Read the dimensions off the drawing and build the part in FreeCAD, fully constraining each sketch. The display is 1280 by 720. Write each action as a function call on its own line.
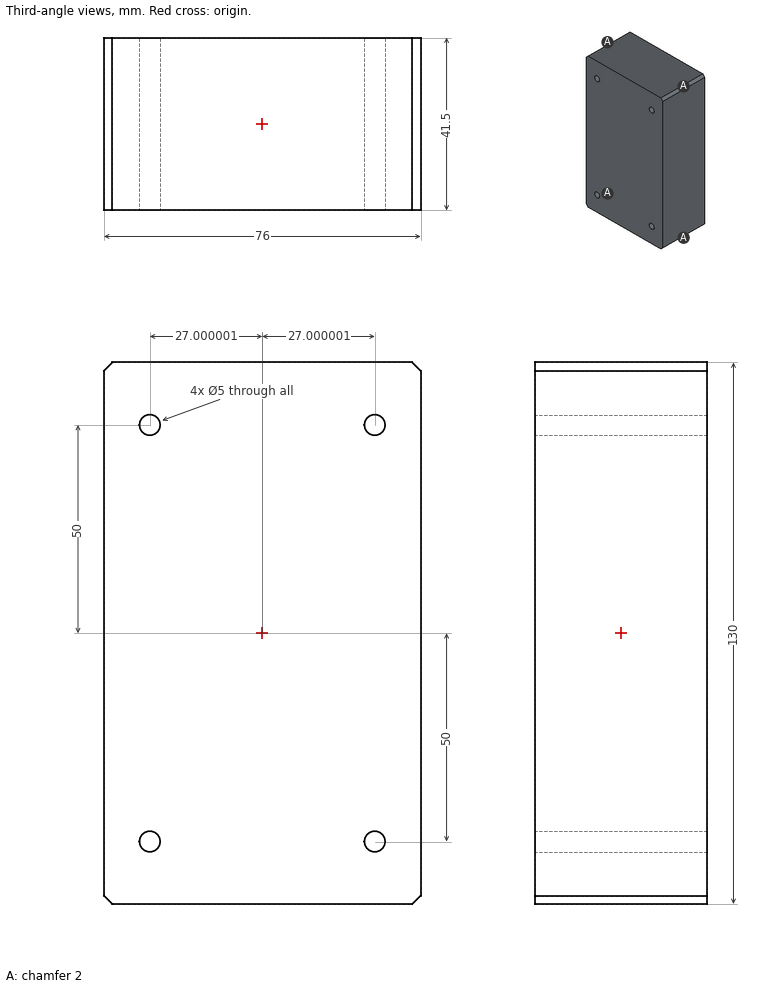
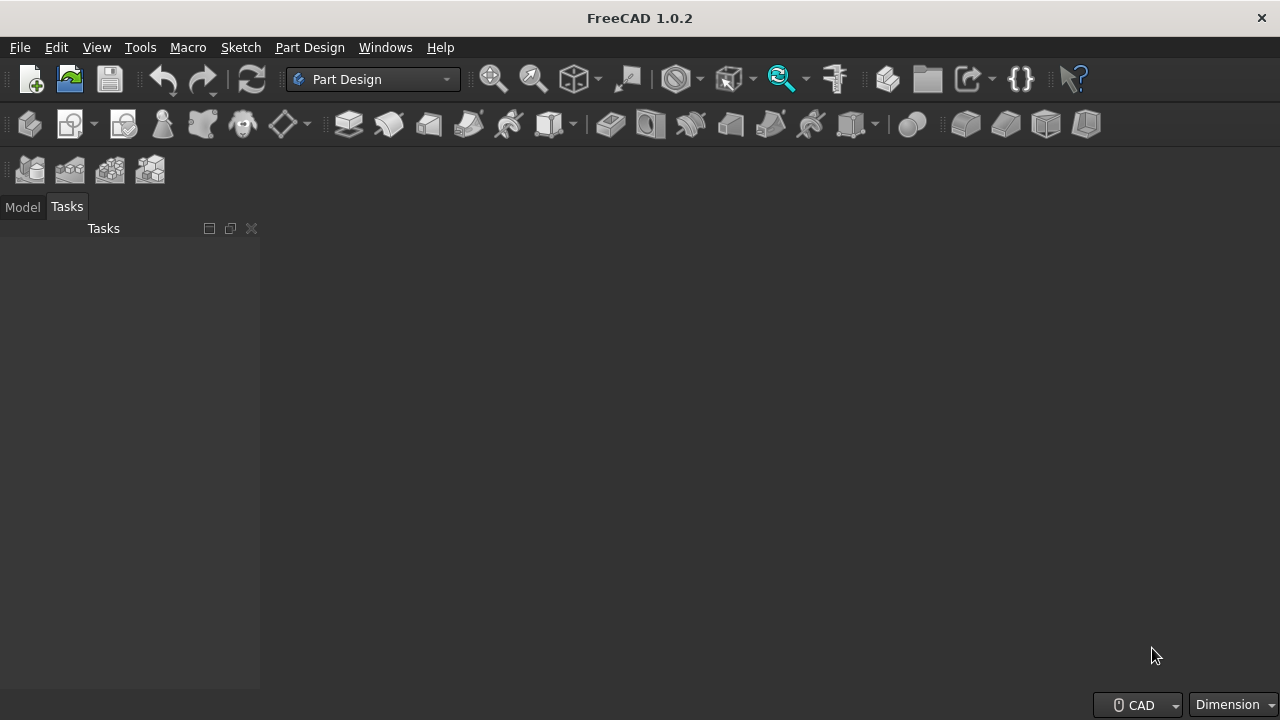
click(30, 80)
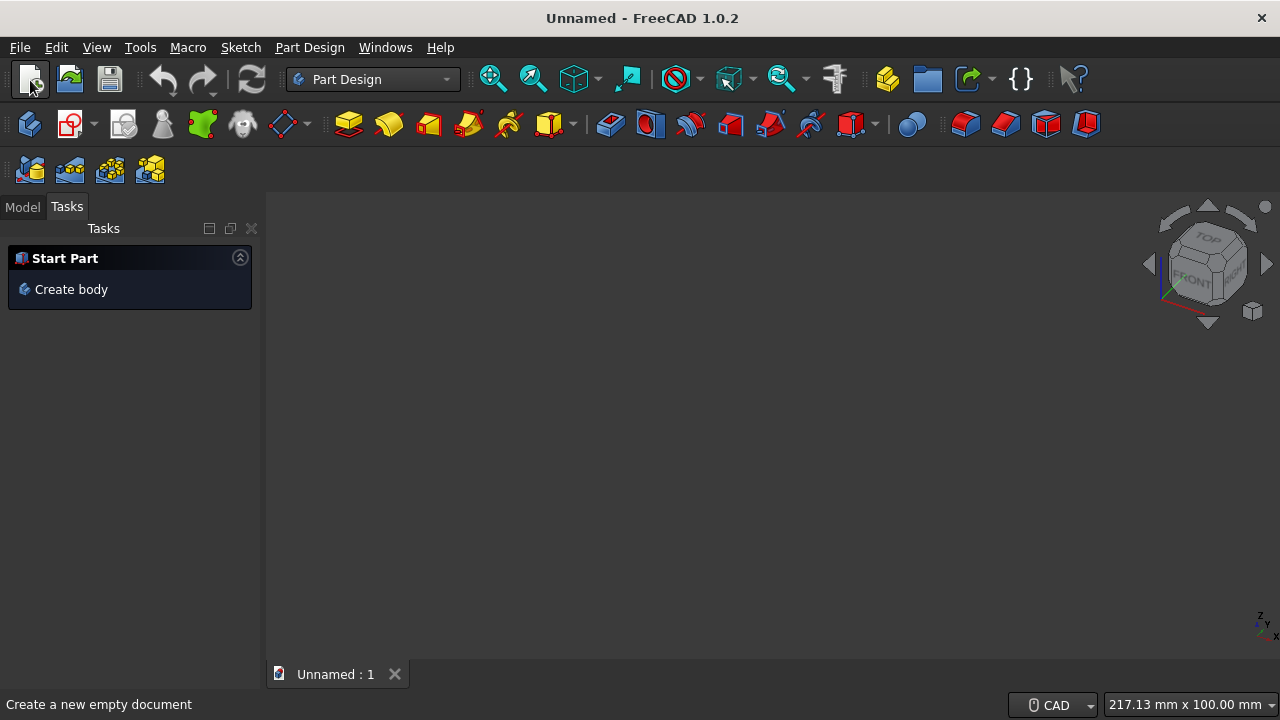
click(70, 124)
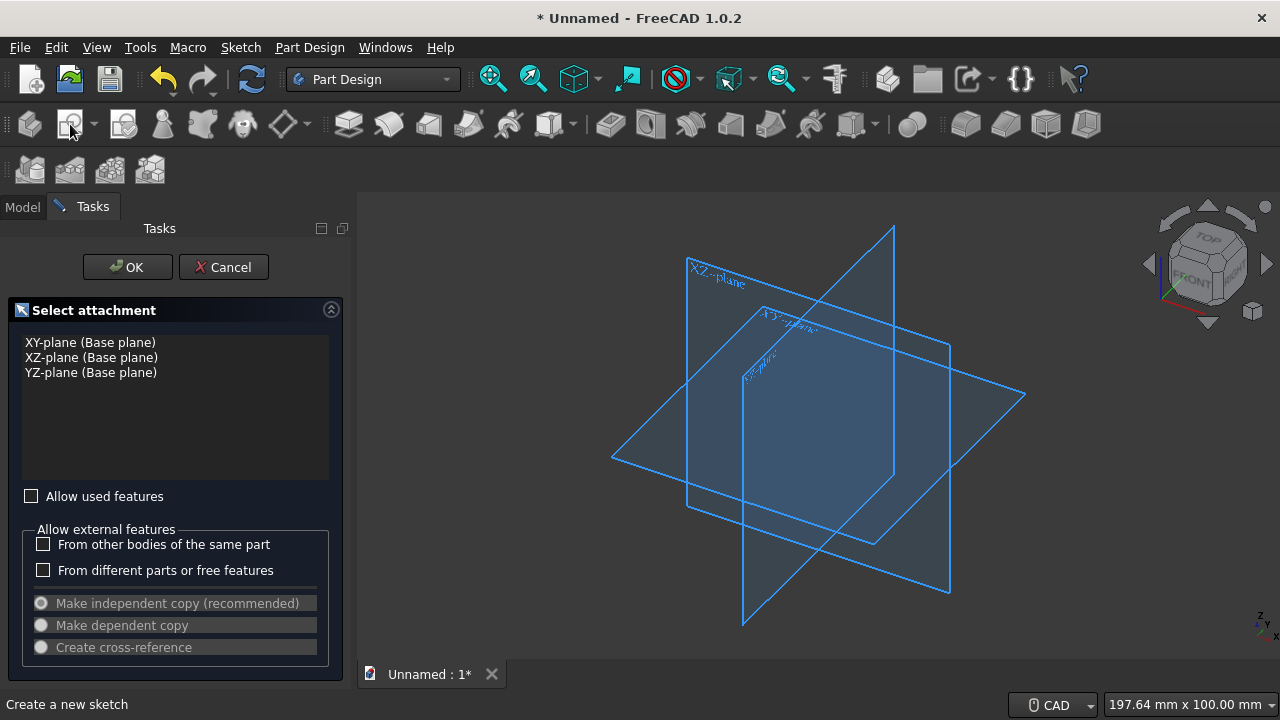
click(82, 342)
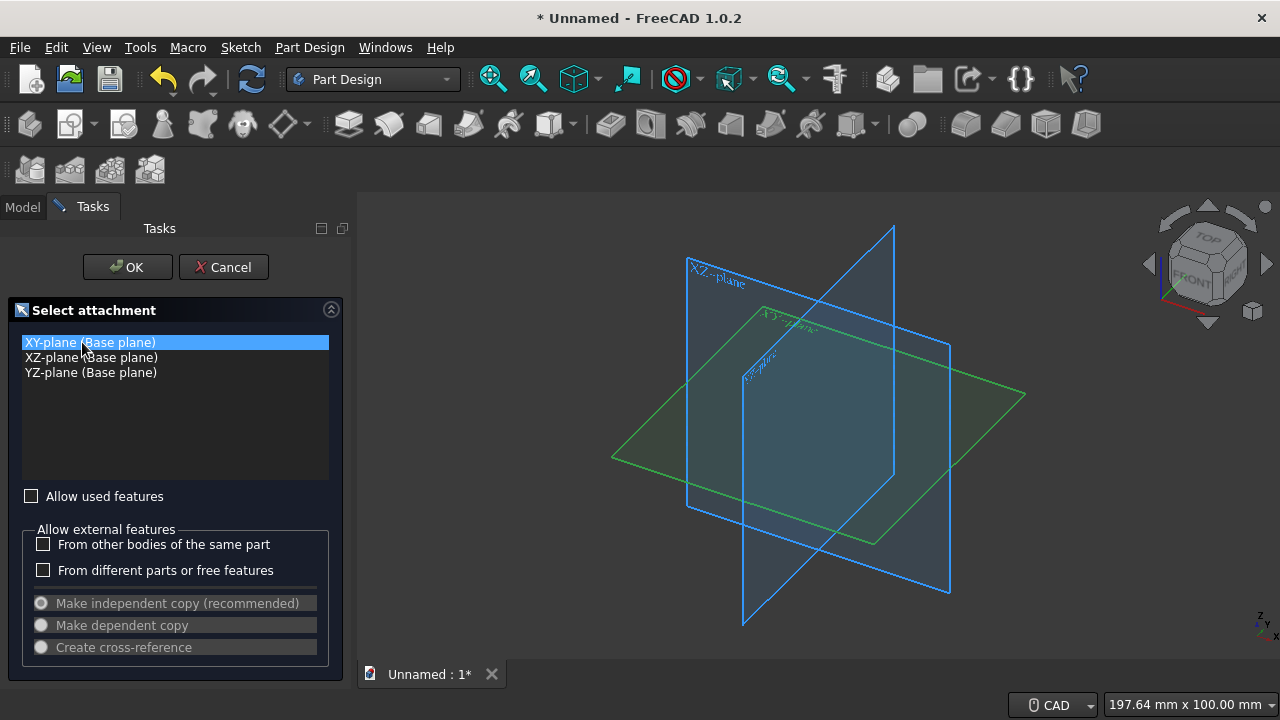
click(128, 267)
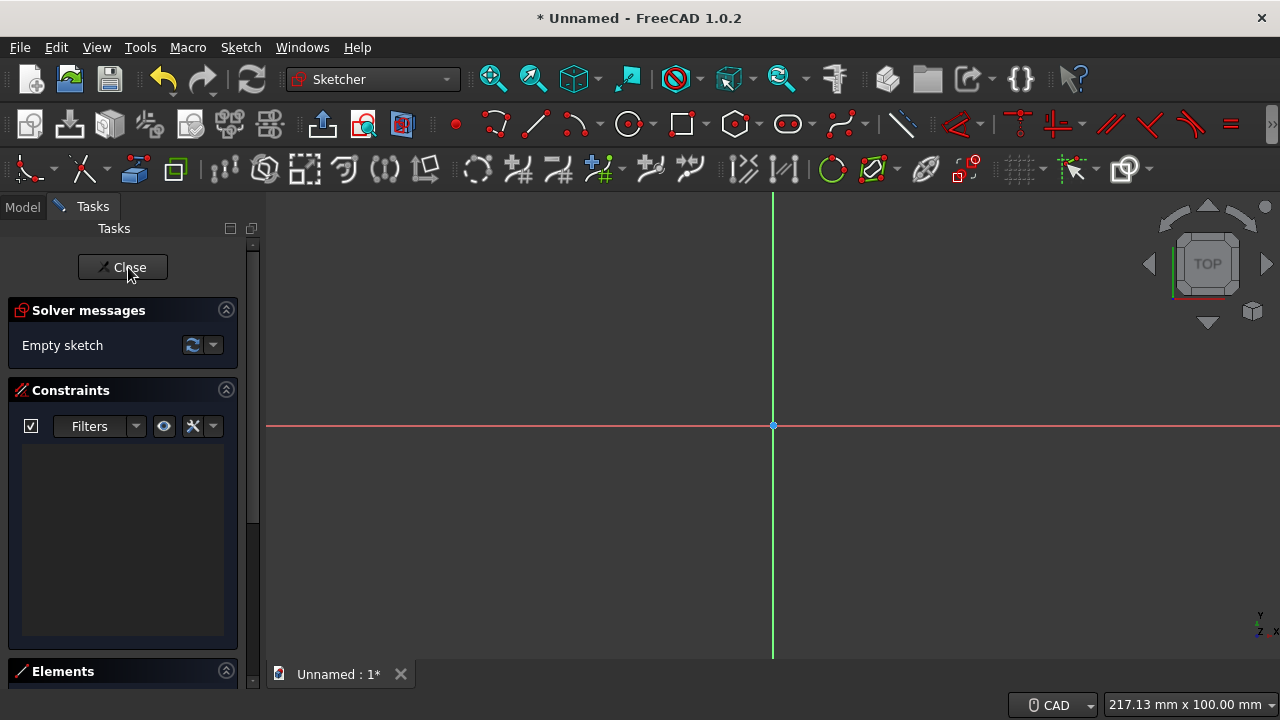
scroll(912, 425, up, 2)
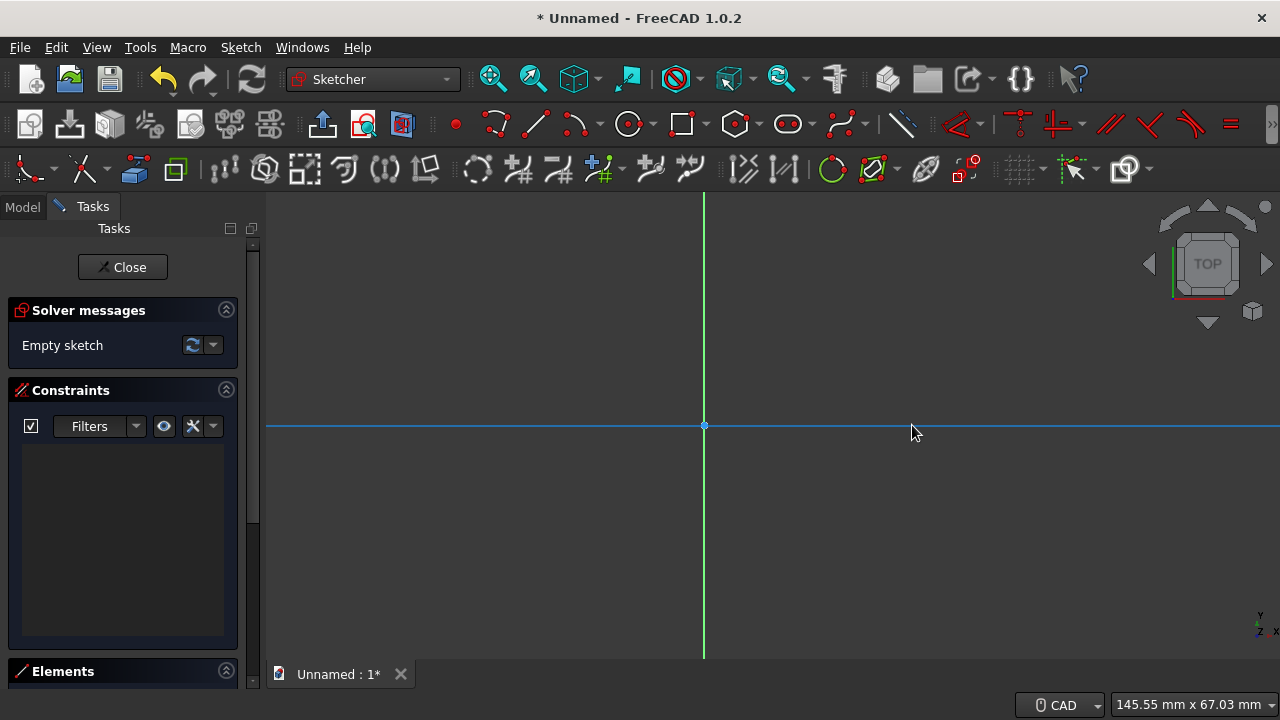
click(708, 124)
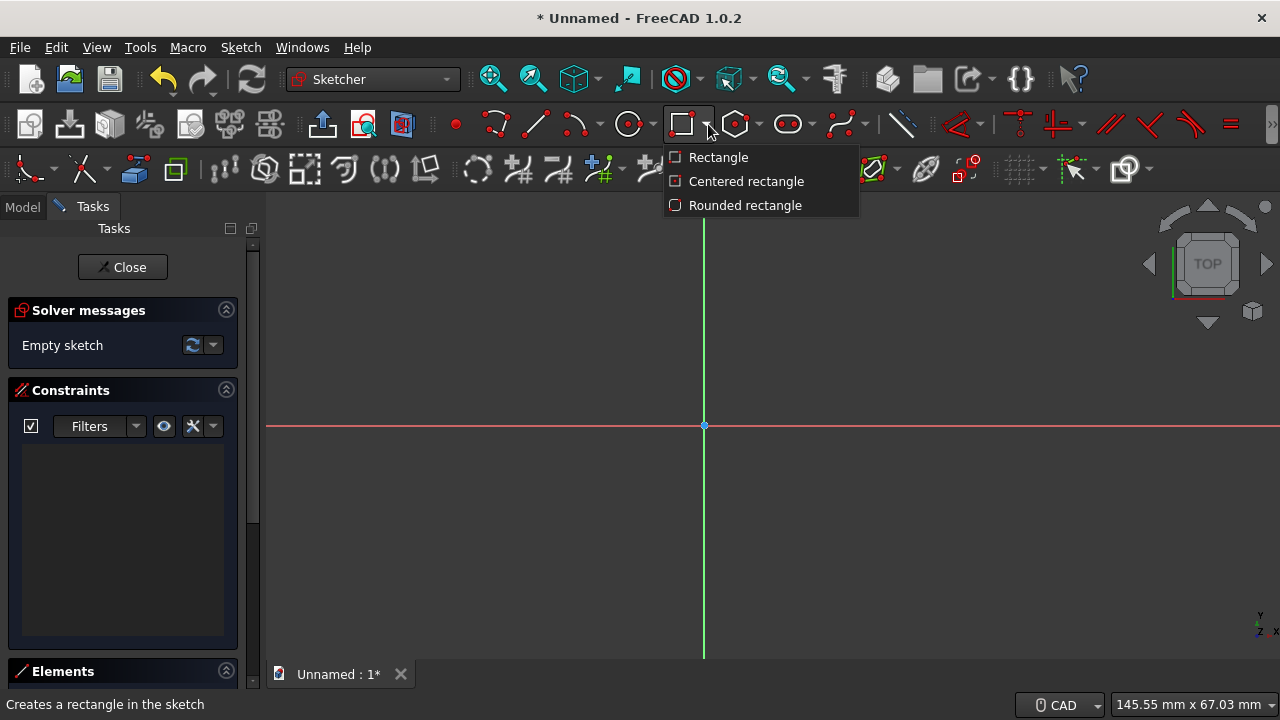
click(762, 181)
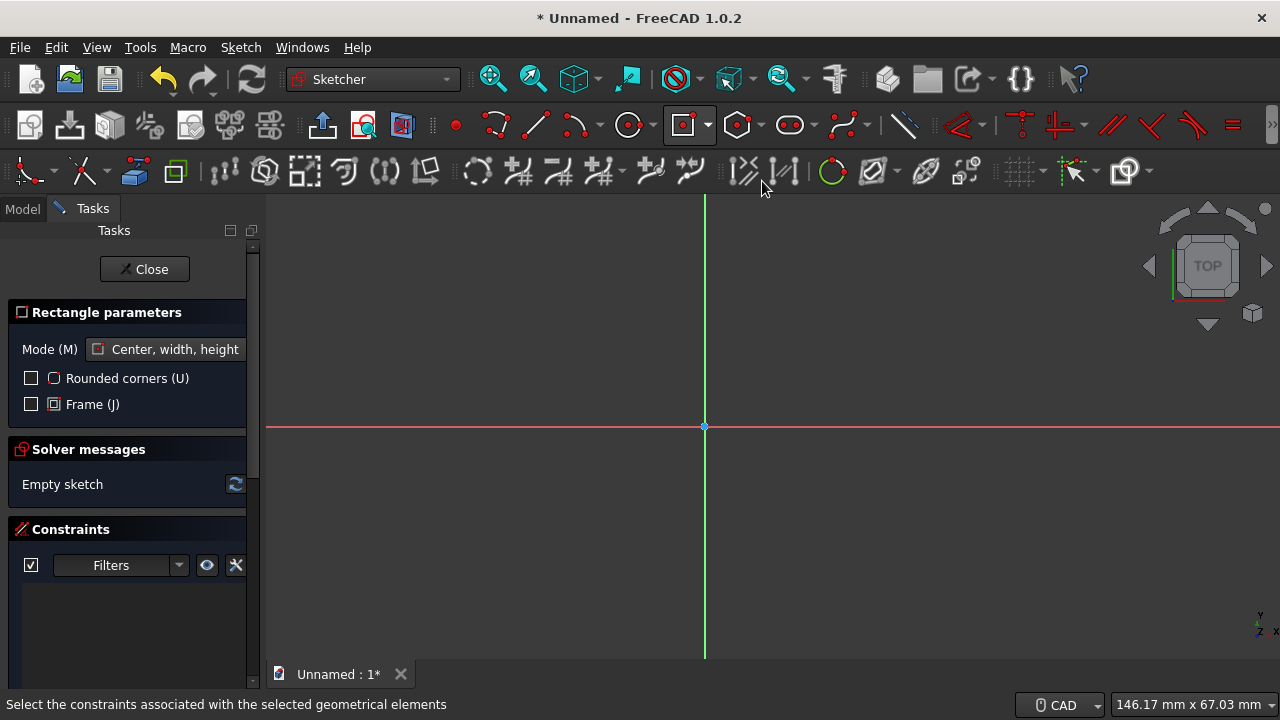
click(705, 426)
move(968, 283)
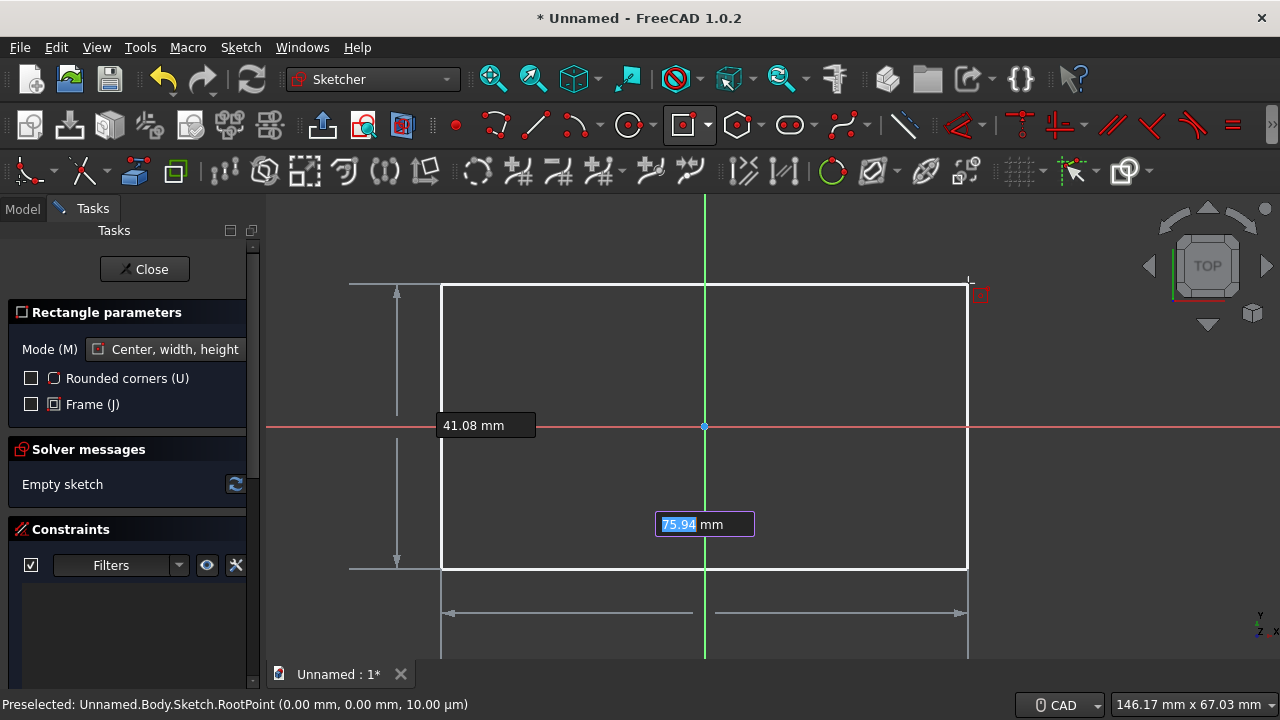
text(76)
key(Tab)
text(41.5)
key(Return)
key(Escape)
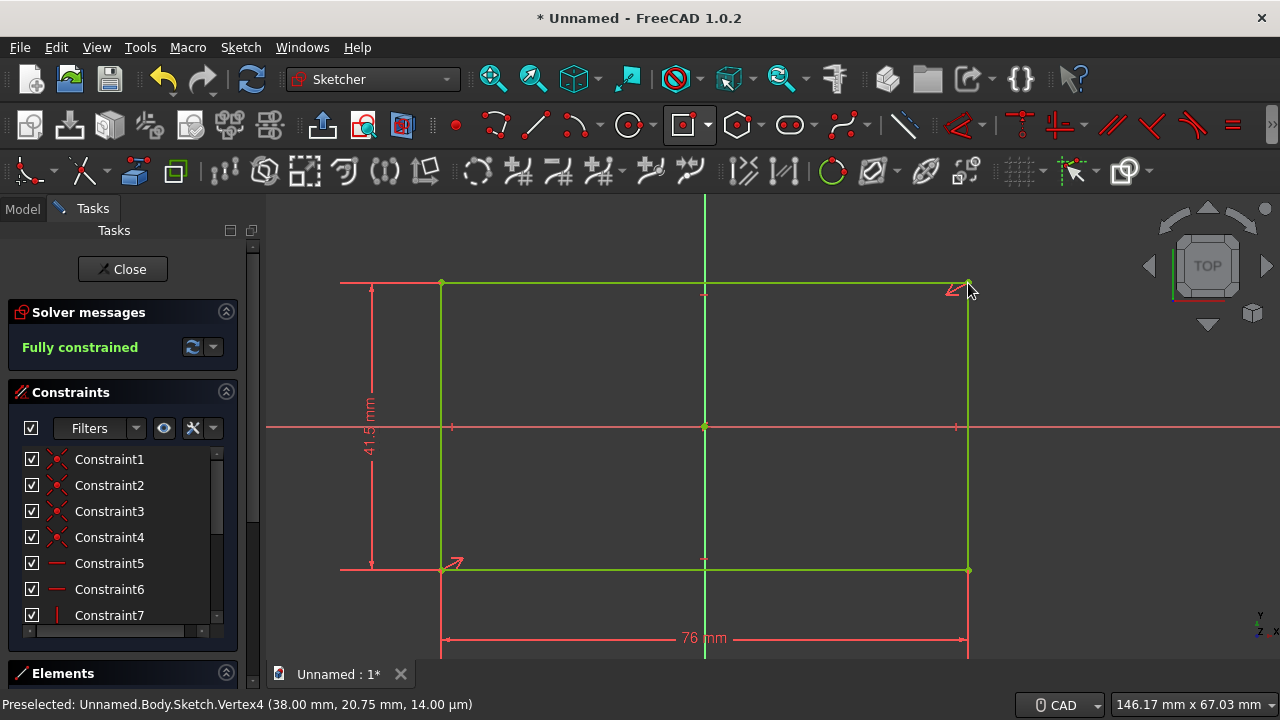
click(123, 269)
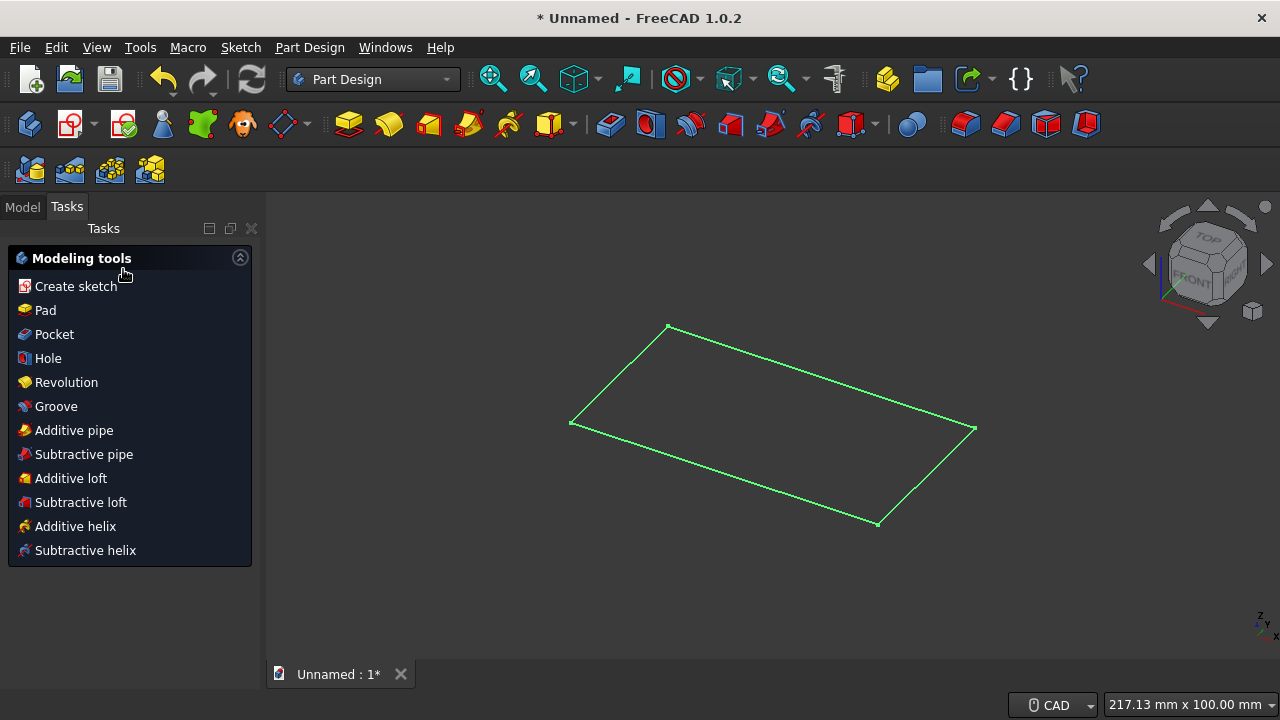
click(350, 124)